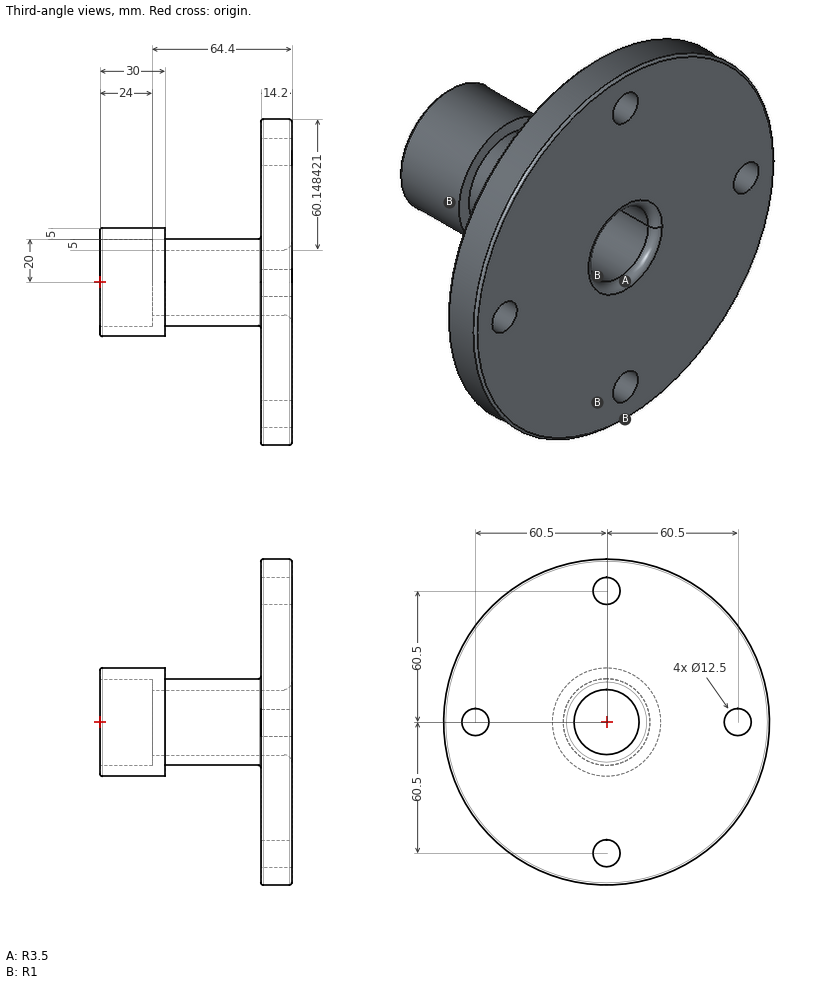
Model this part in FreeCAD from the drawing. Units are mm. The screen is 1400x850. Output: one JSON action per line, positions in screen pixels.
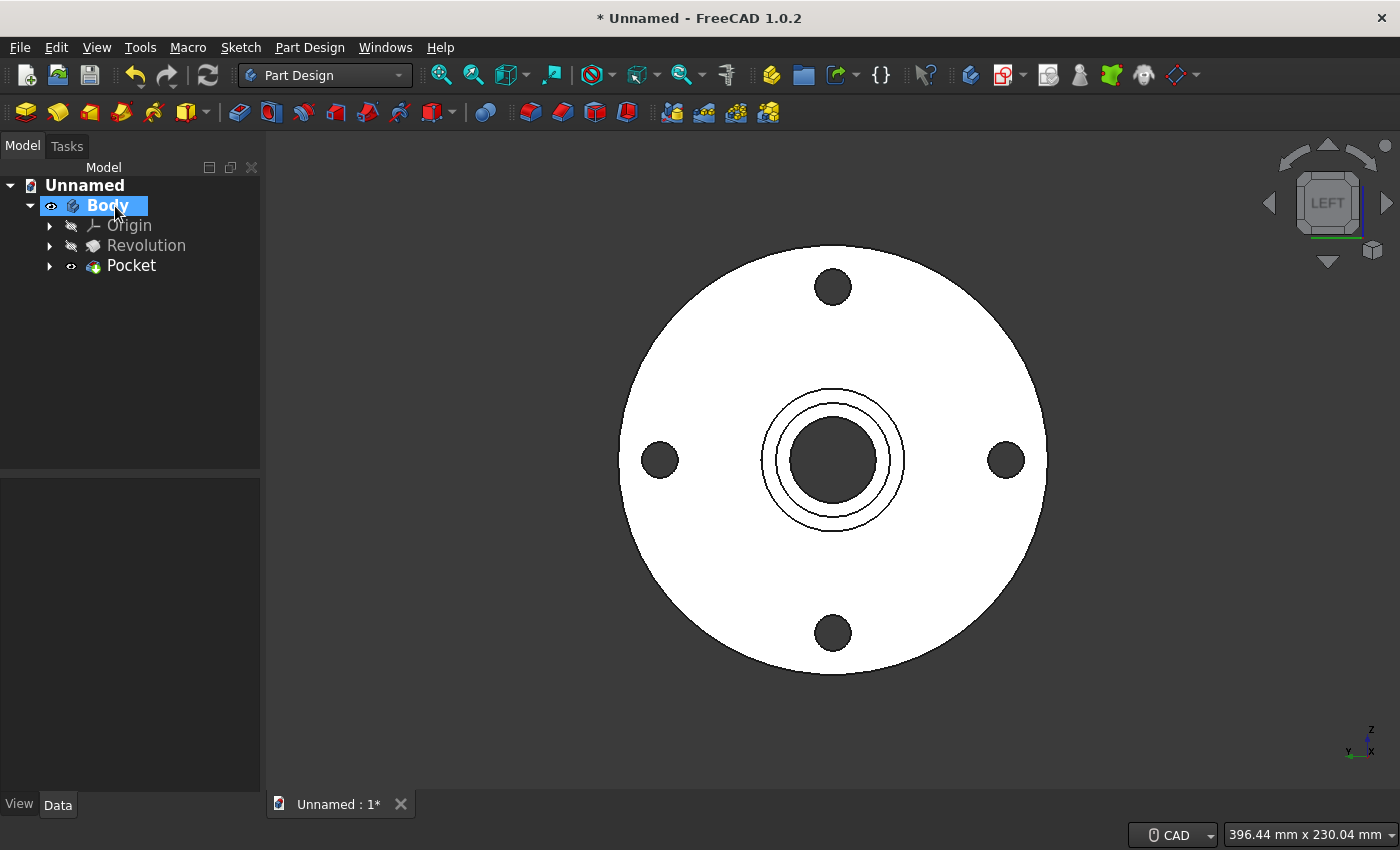
{"action": "key", "text": "0"}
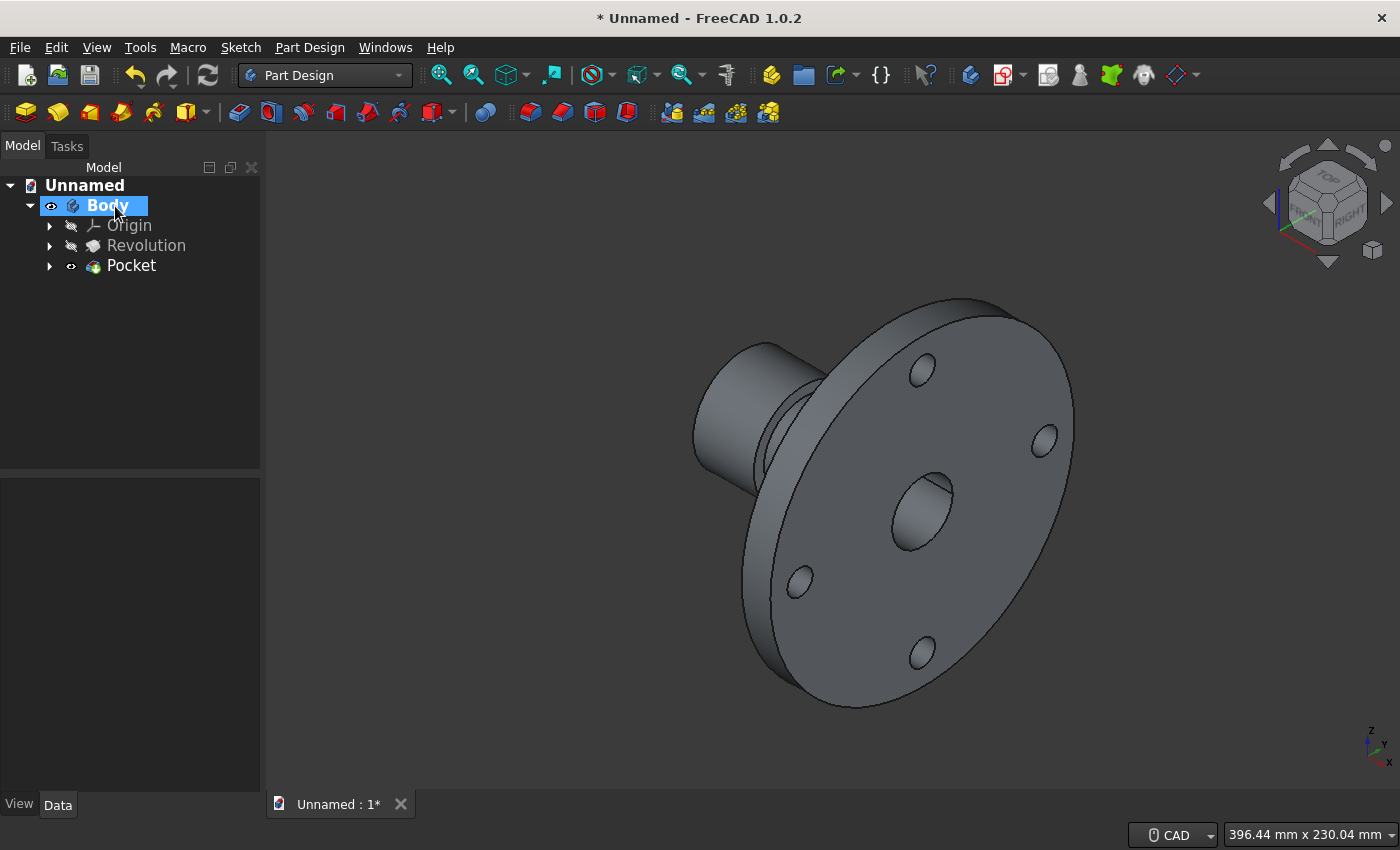
{"action": "left_click", "coordinate": [913, 549]}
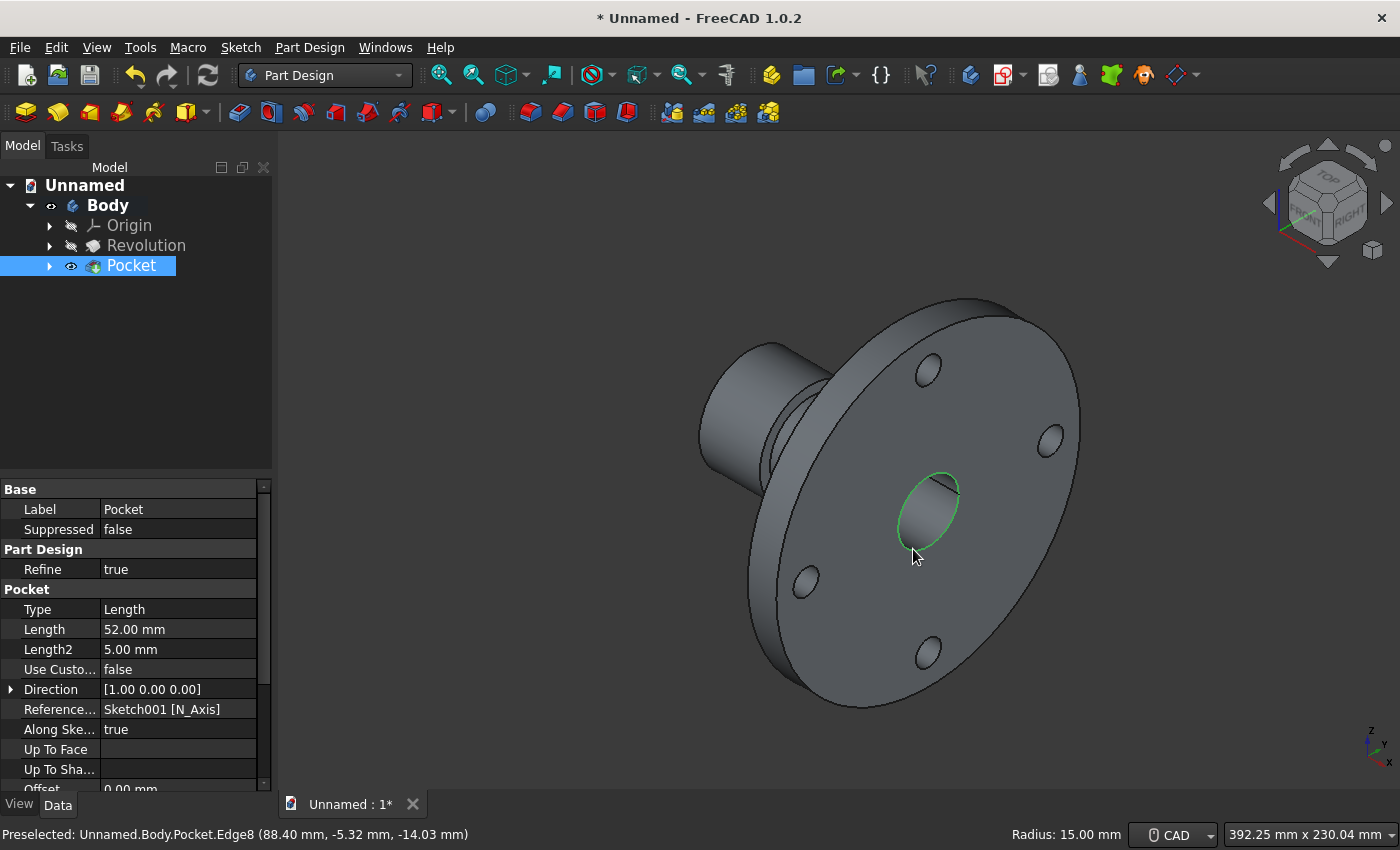
{"action": "left_click", "coordinate": [532, 112]}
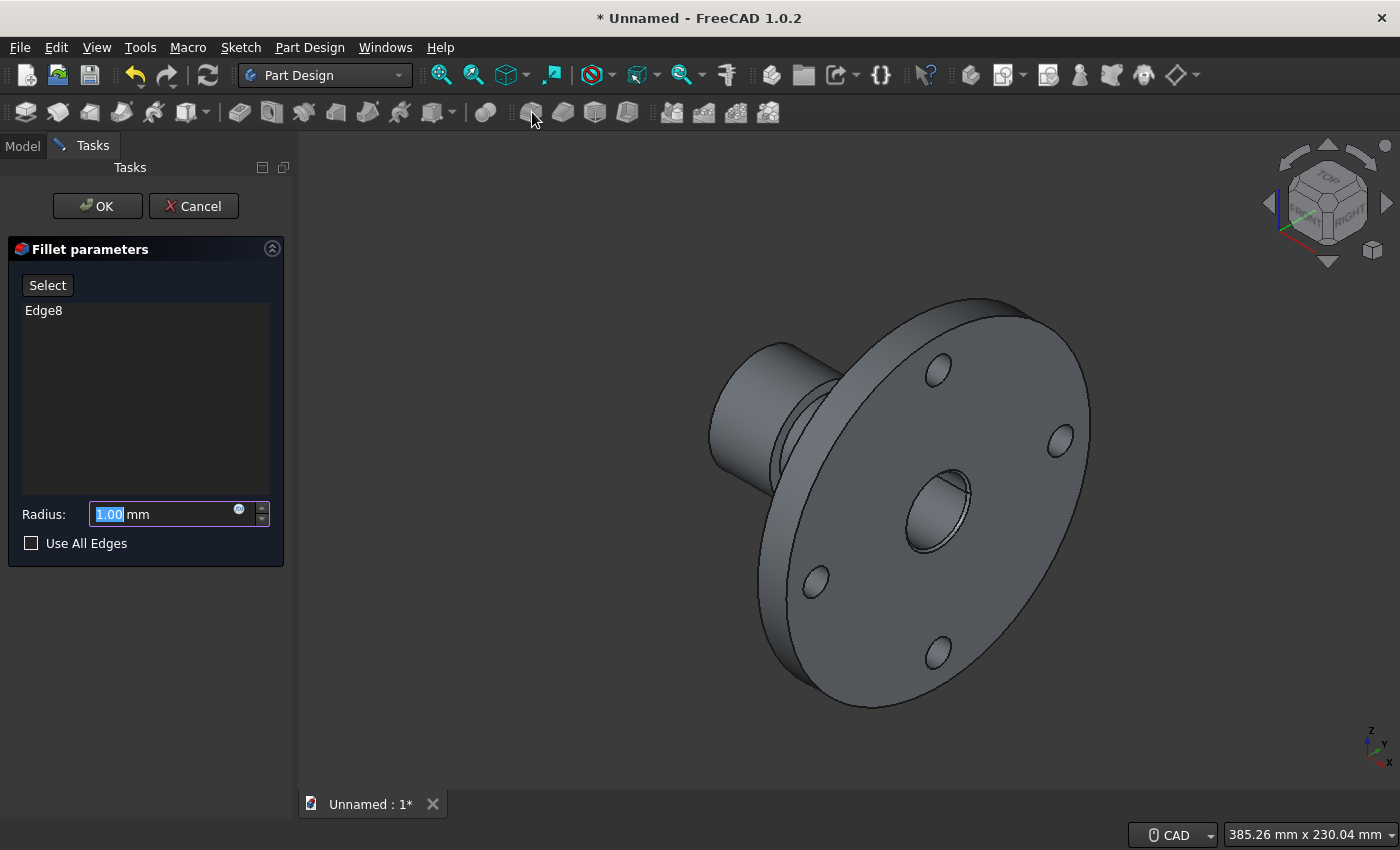
{"action": "type", "text": "3.5"}
{"action": "key", "text": "Tab"}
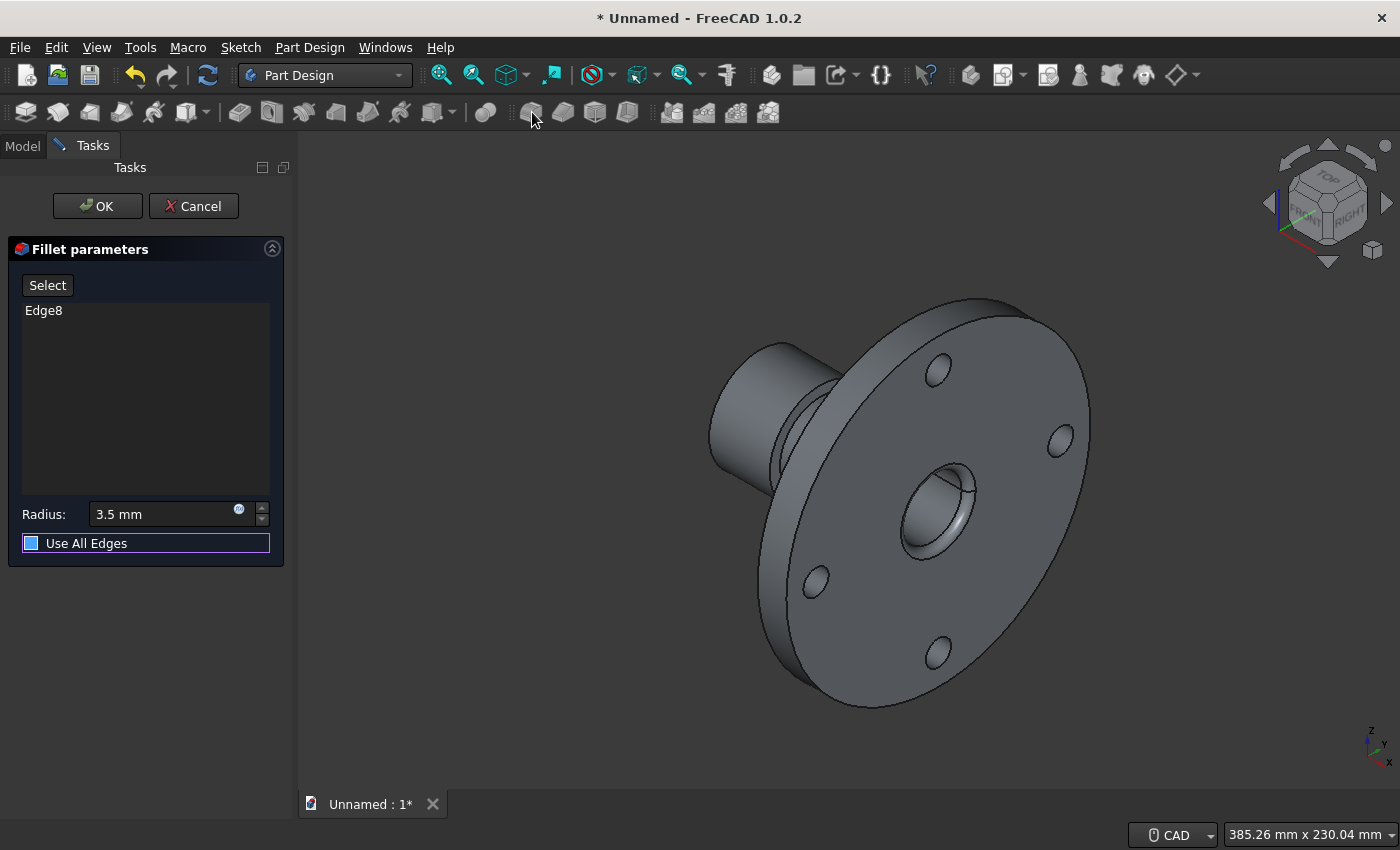
{"action": "left_click", "coordinate": [98, 206]}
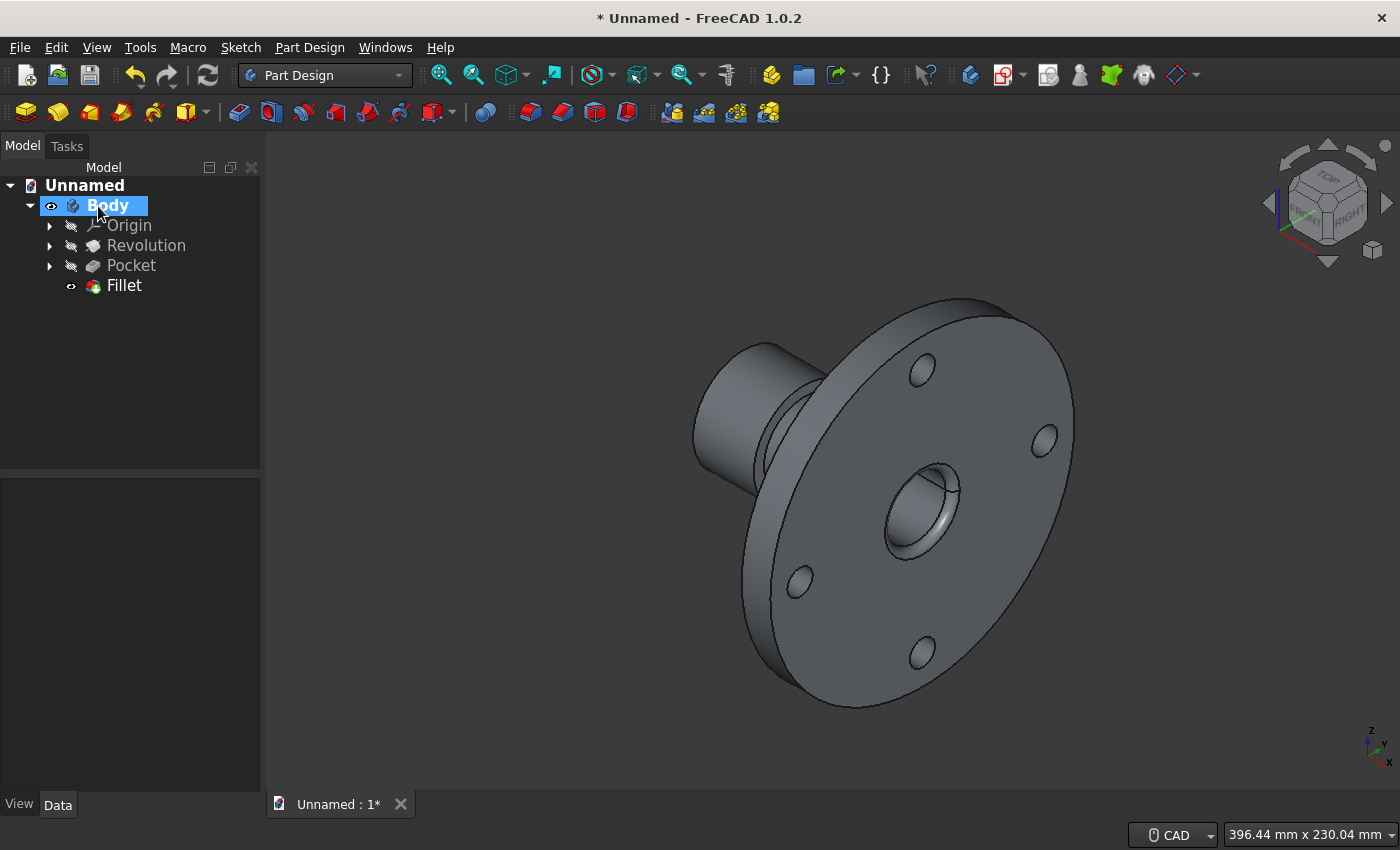
{"action": "left_click", "coordinate": [770, 598]}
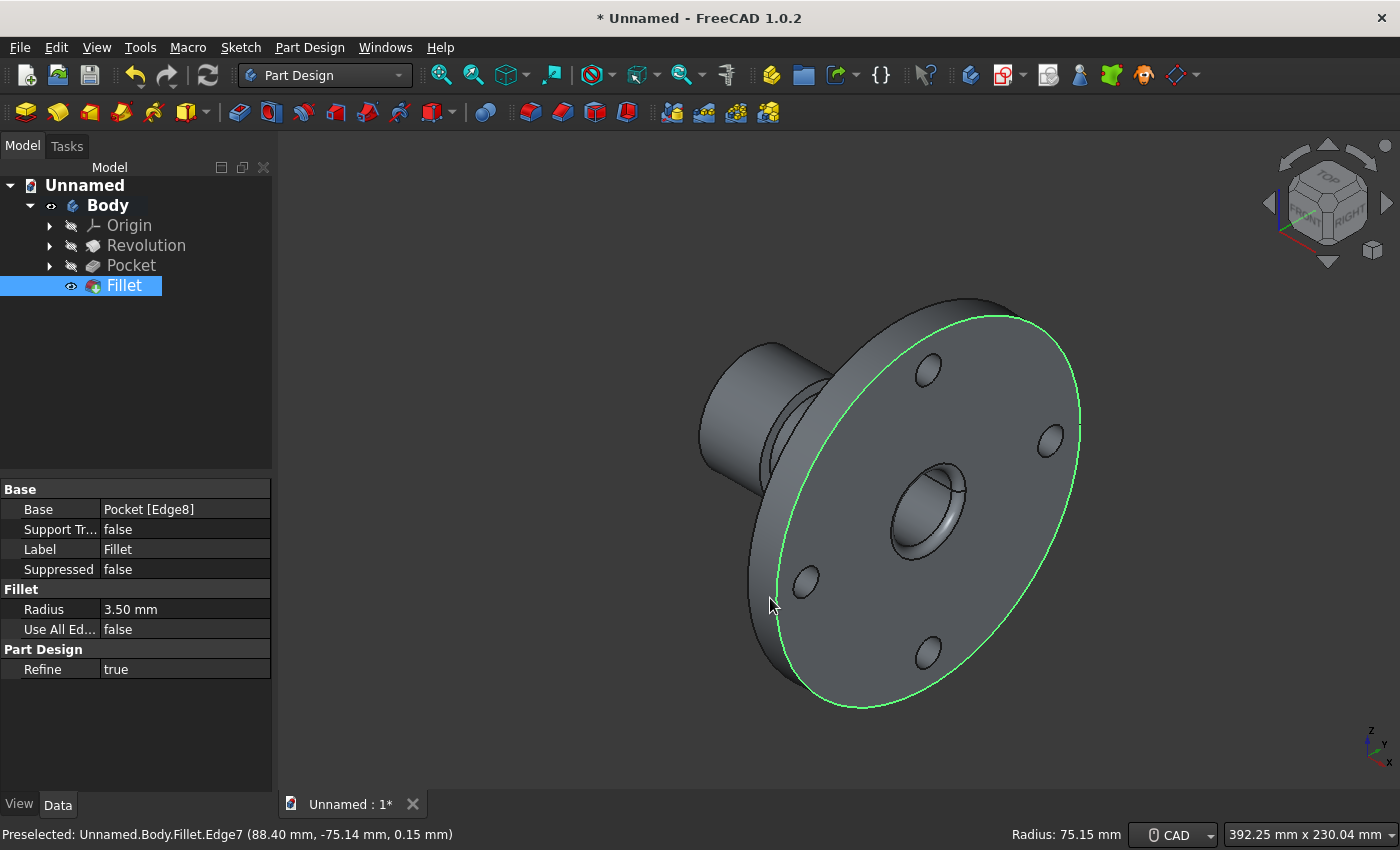
{"action": "key", "text": "2"}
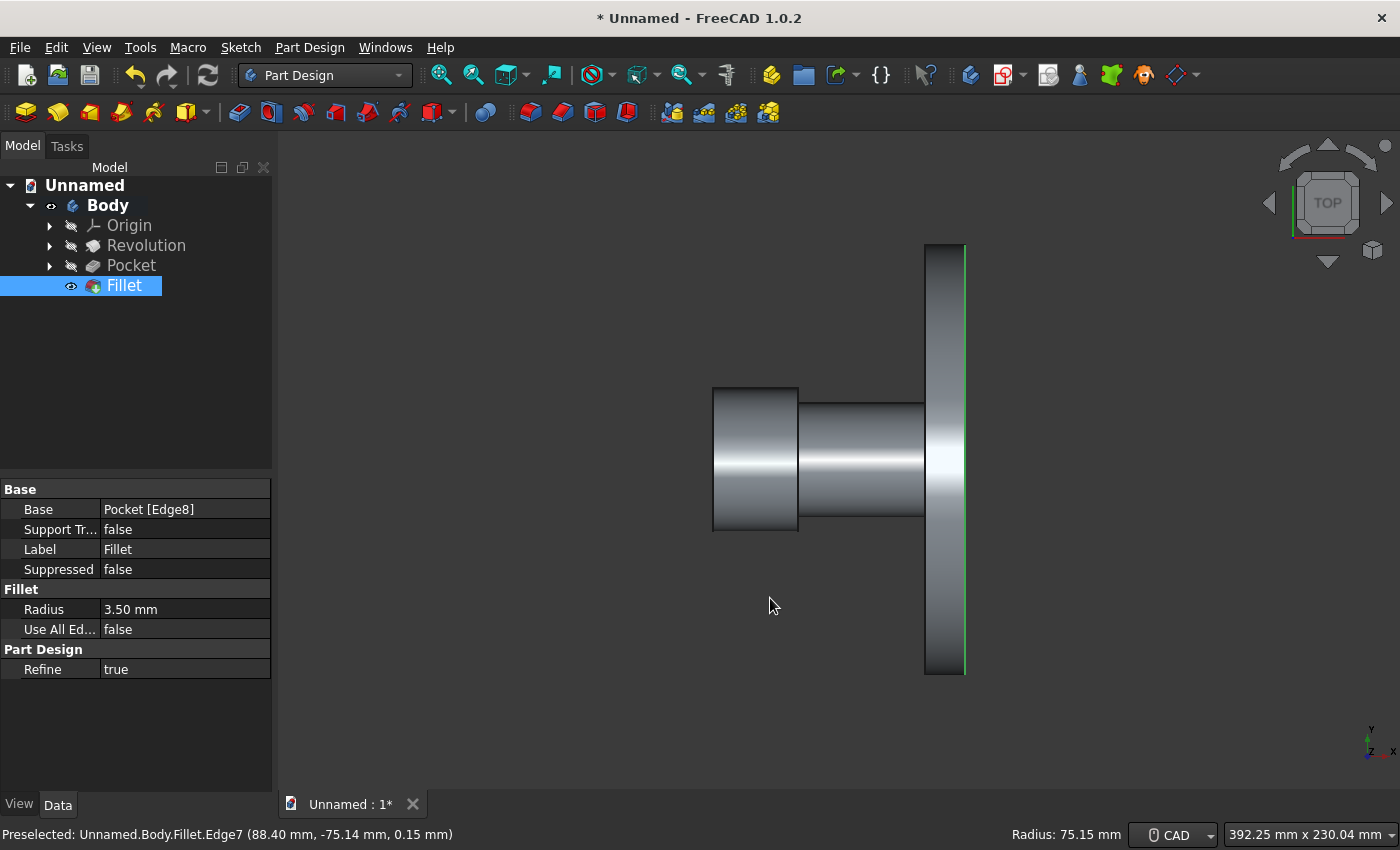
{"action": "left_click", "coordinate": [925, 633], "text": "ctrl"}